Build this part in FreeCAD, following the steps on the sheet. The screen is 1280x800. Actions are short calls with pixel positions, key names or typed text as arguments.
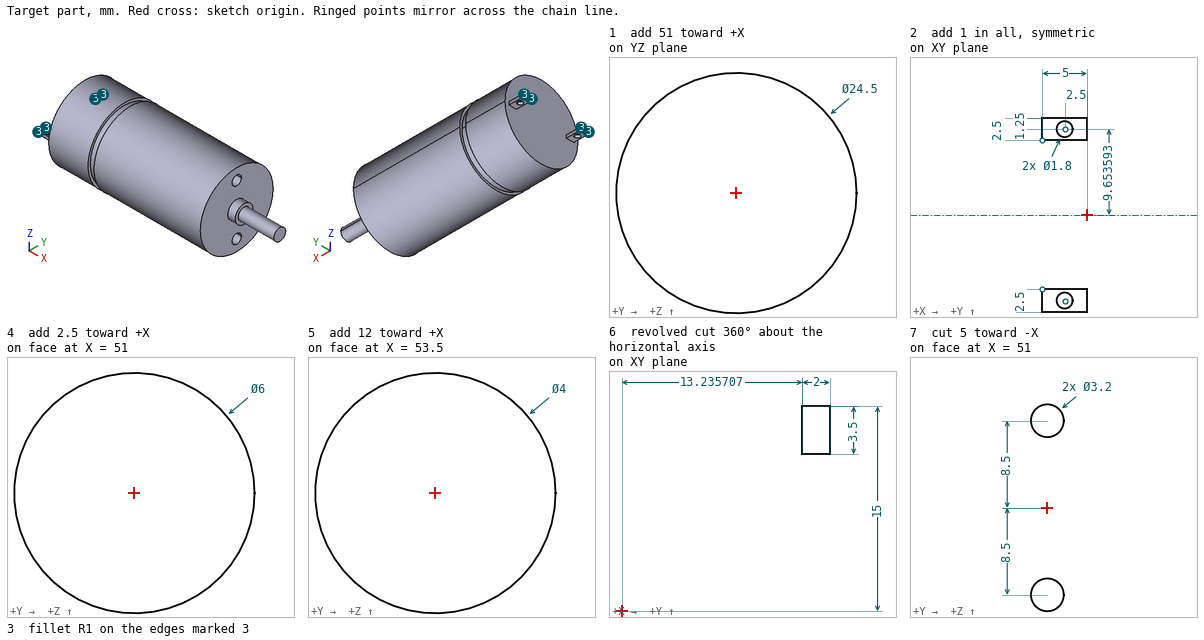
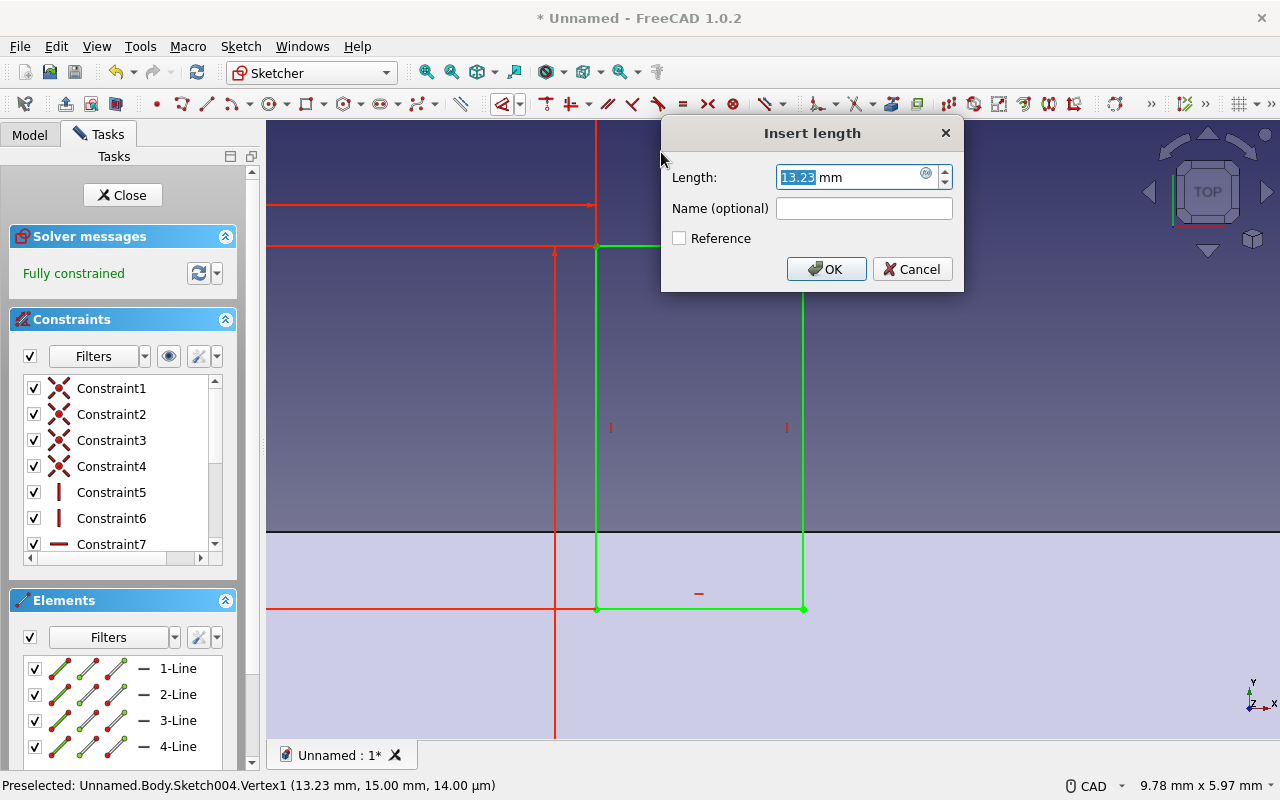
text(13.235707)
key(Return)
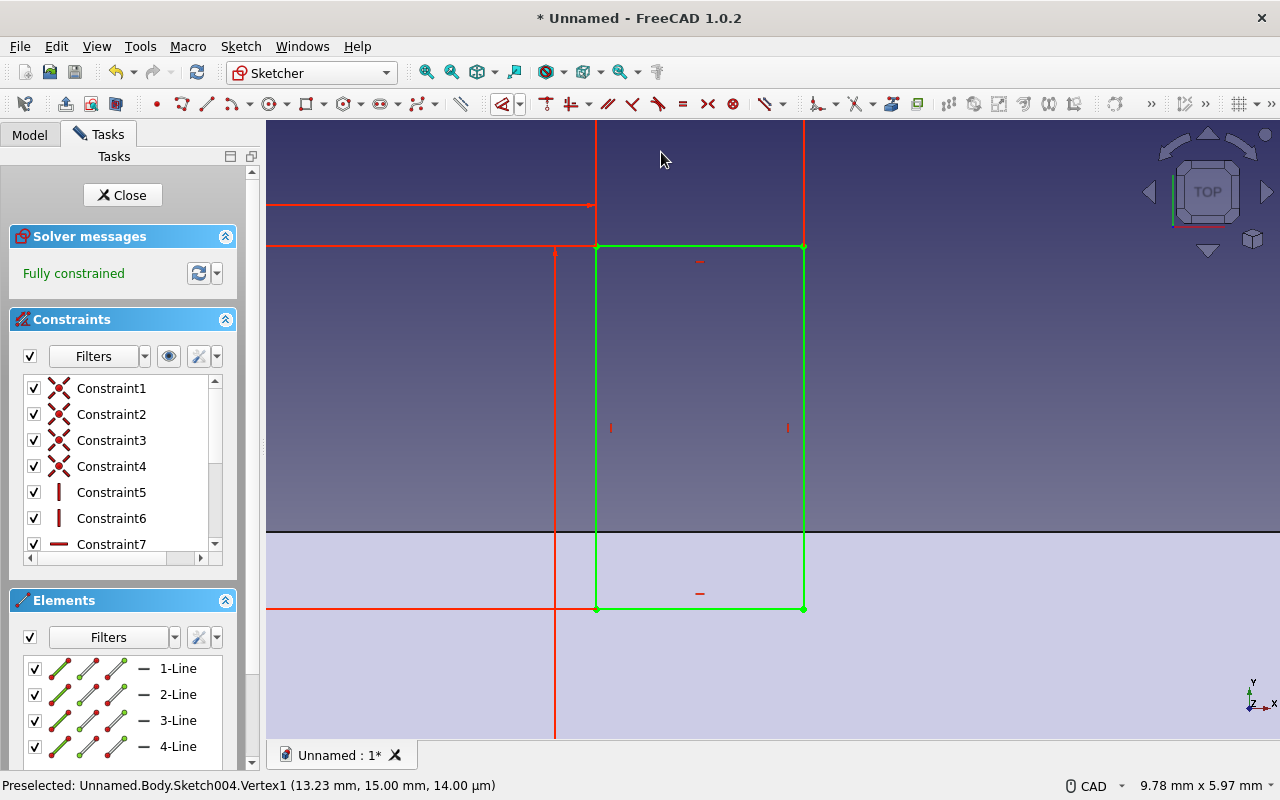
click(123, 195)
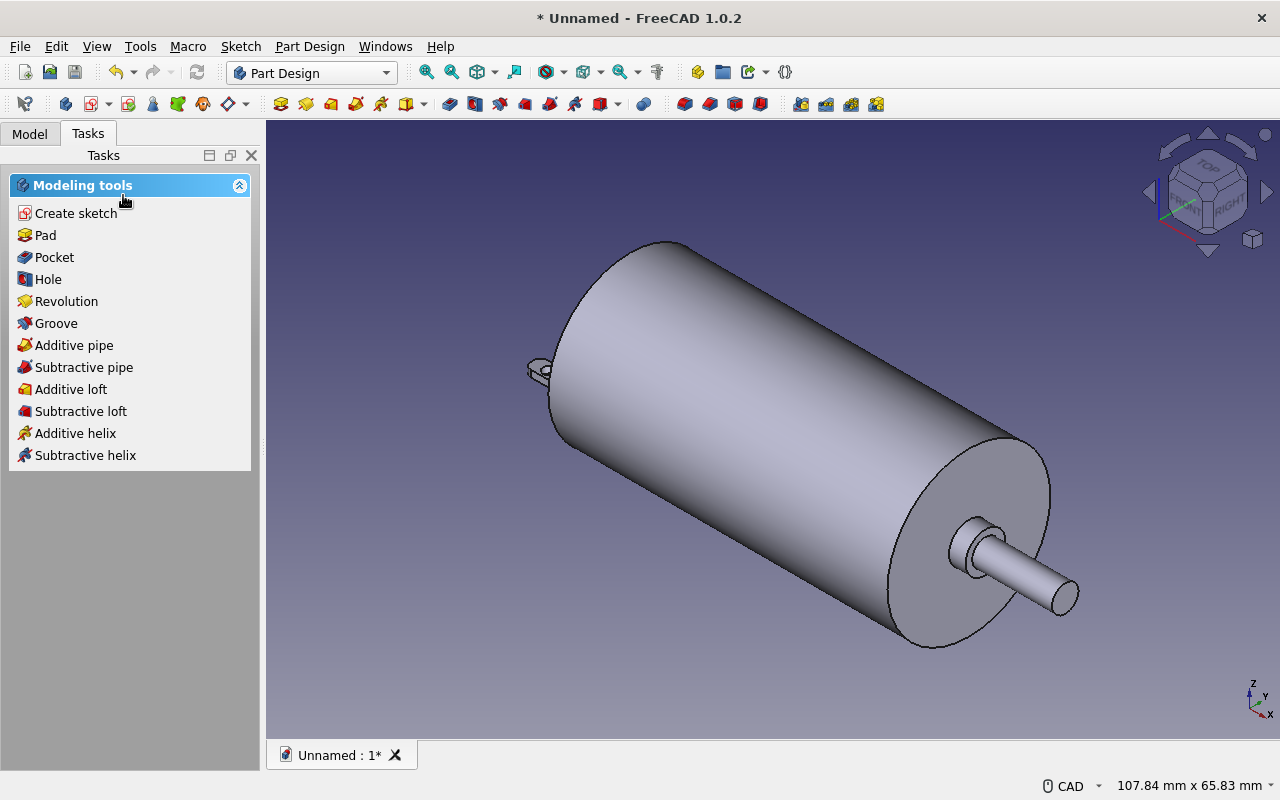
click(500, 104)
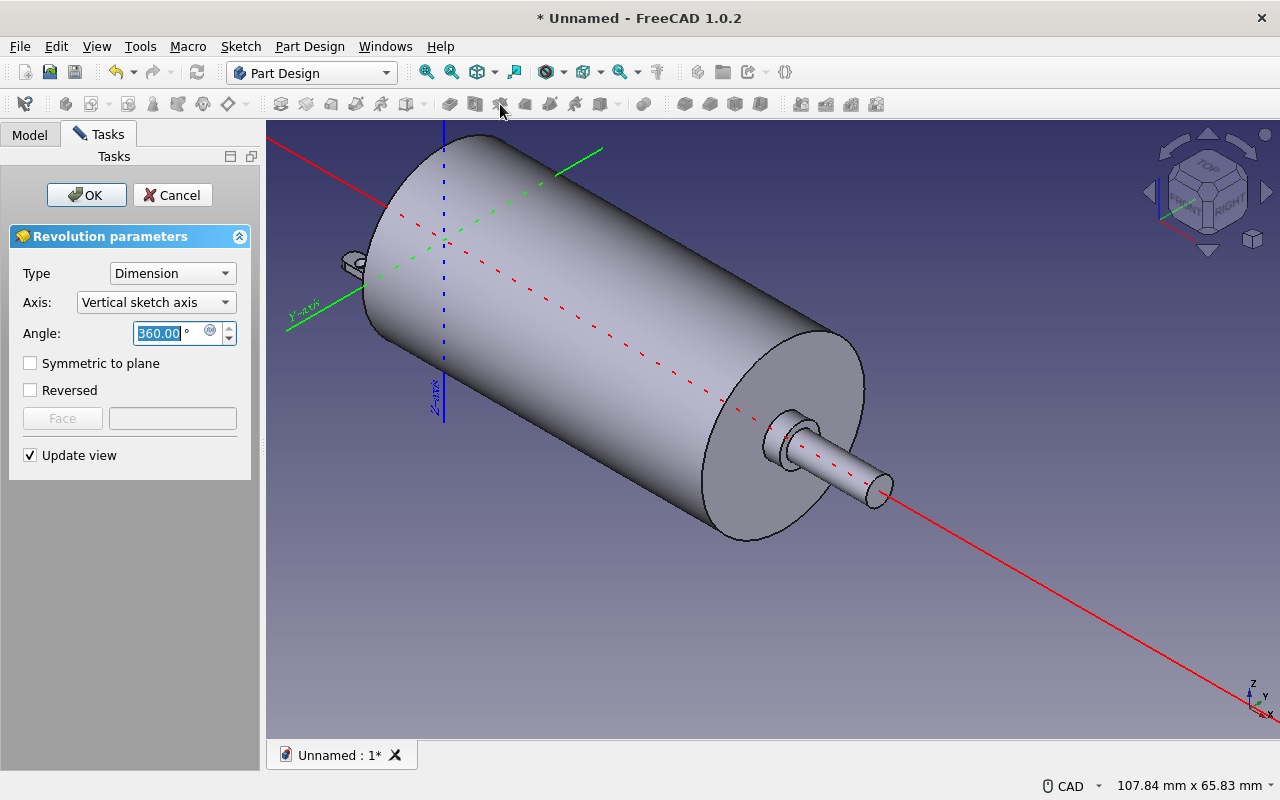
click(157, 302)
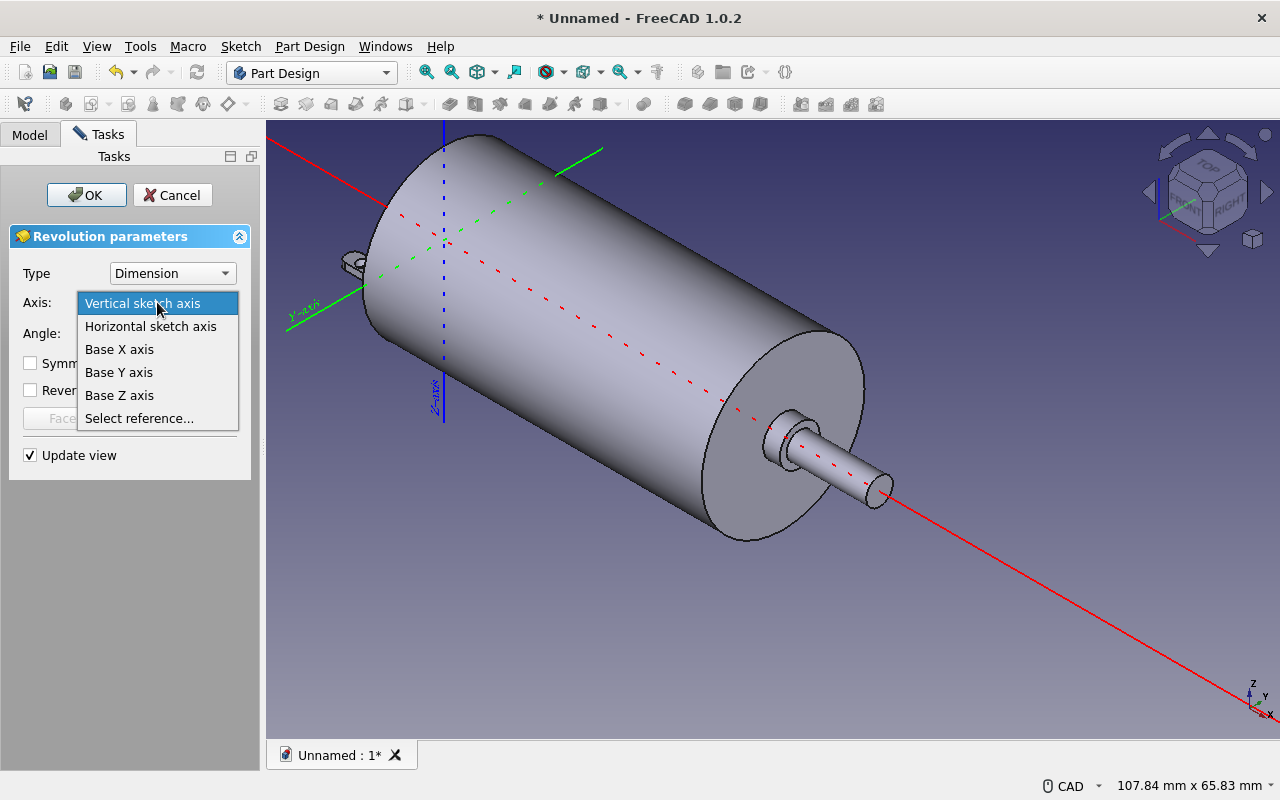
click(156, 326)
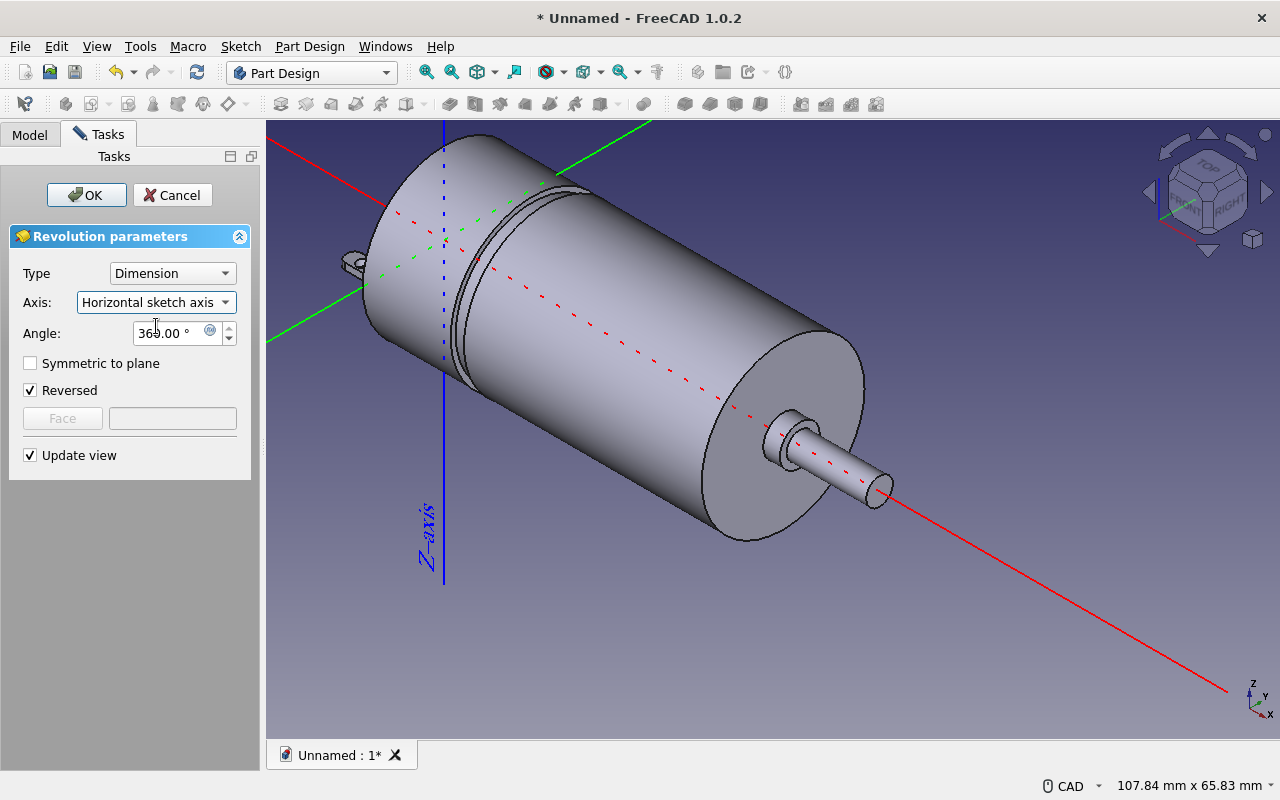
click(87, 195)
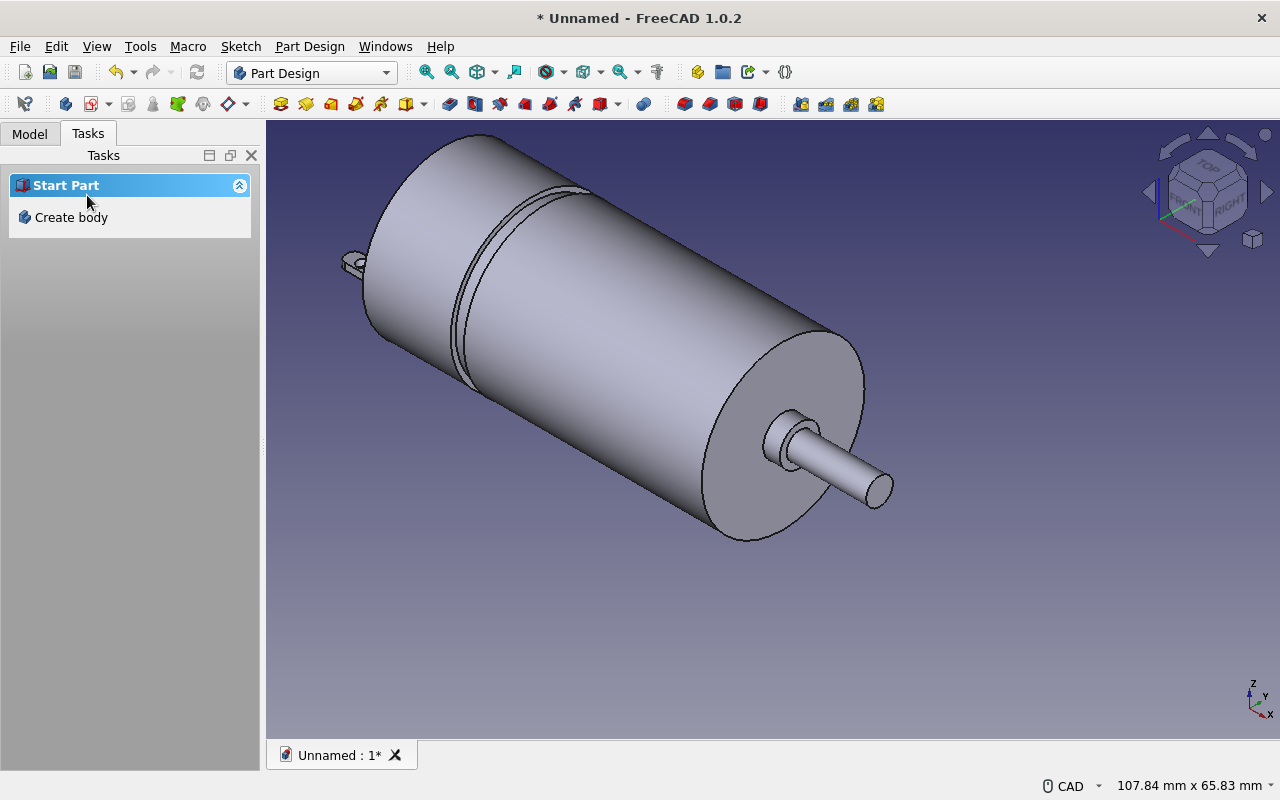
click(427, 72)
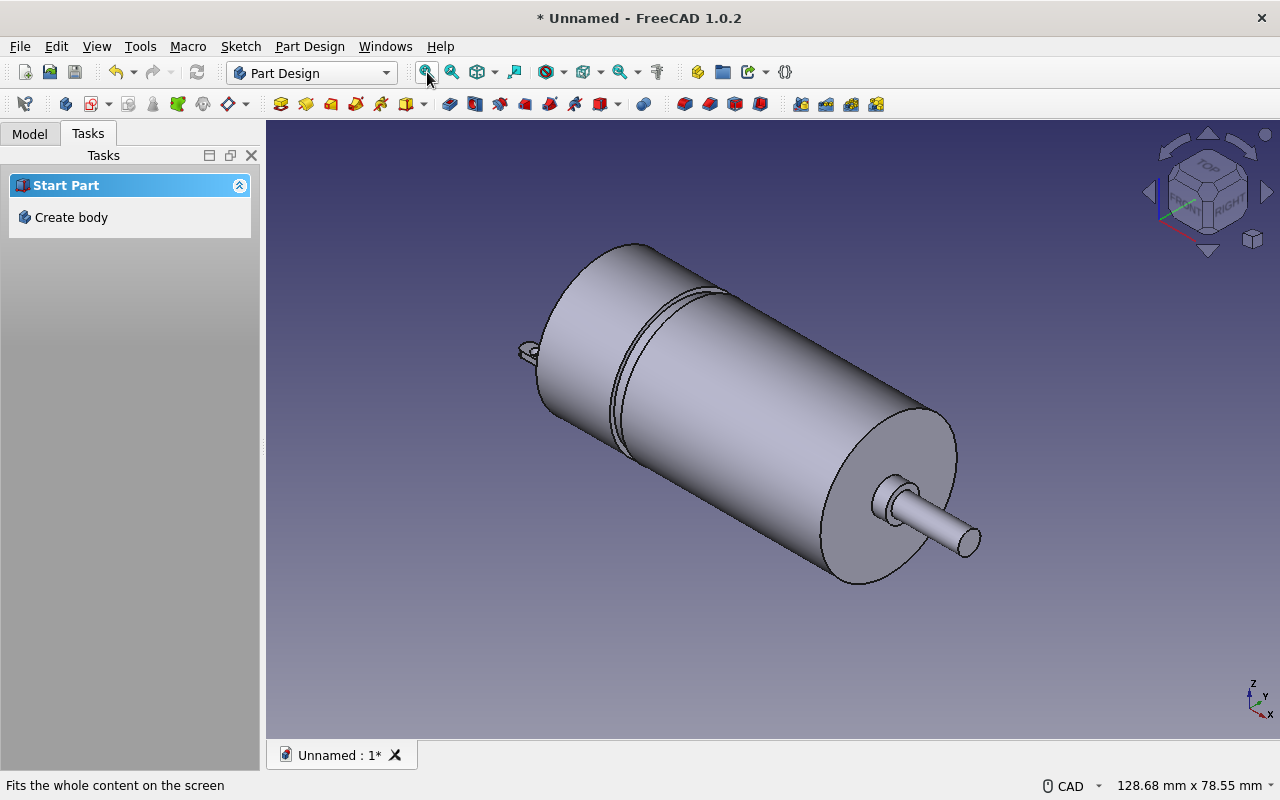
click(869, 461)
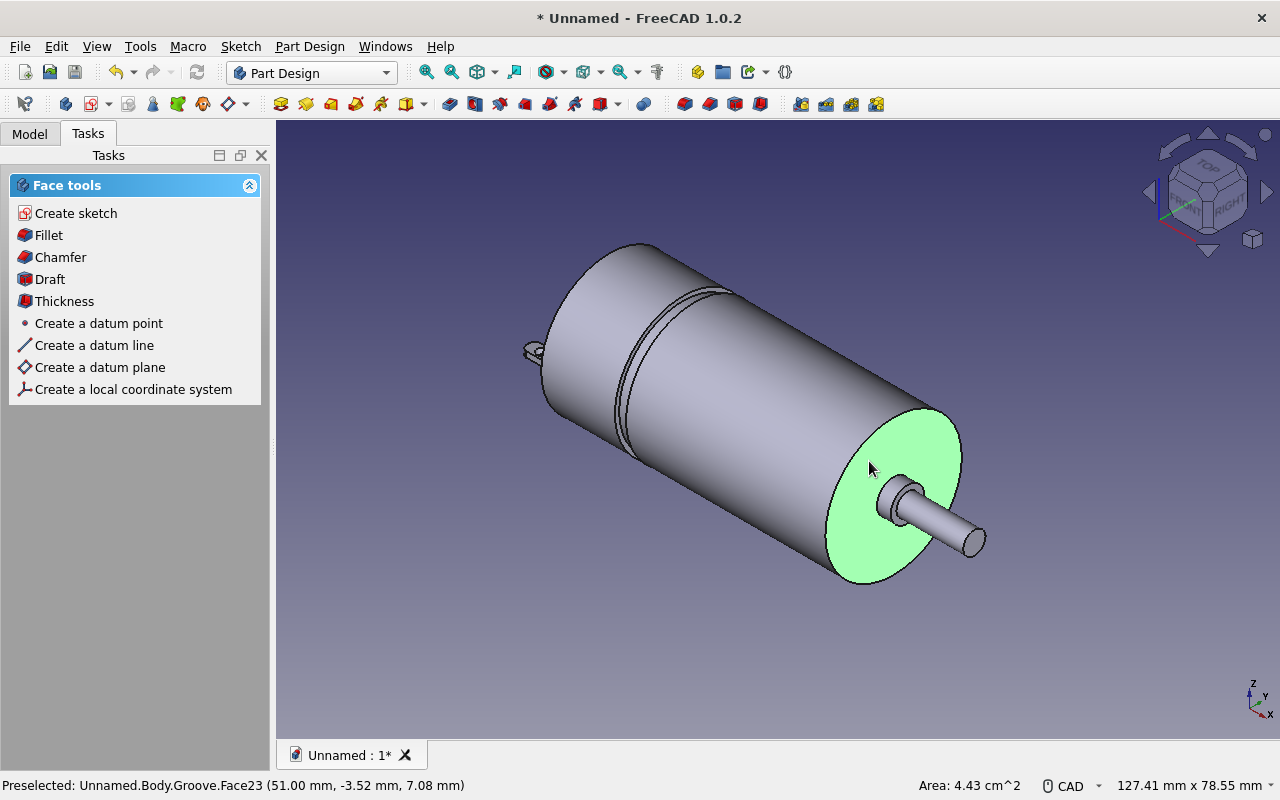
click(90, 104)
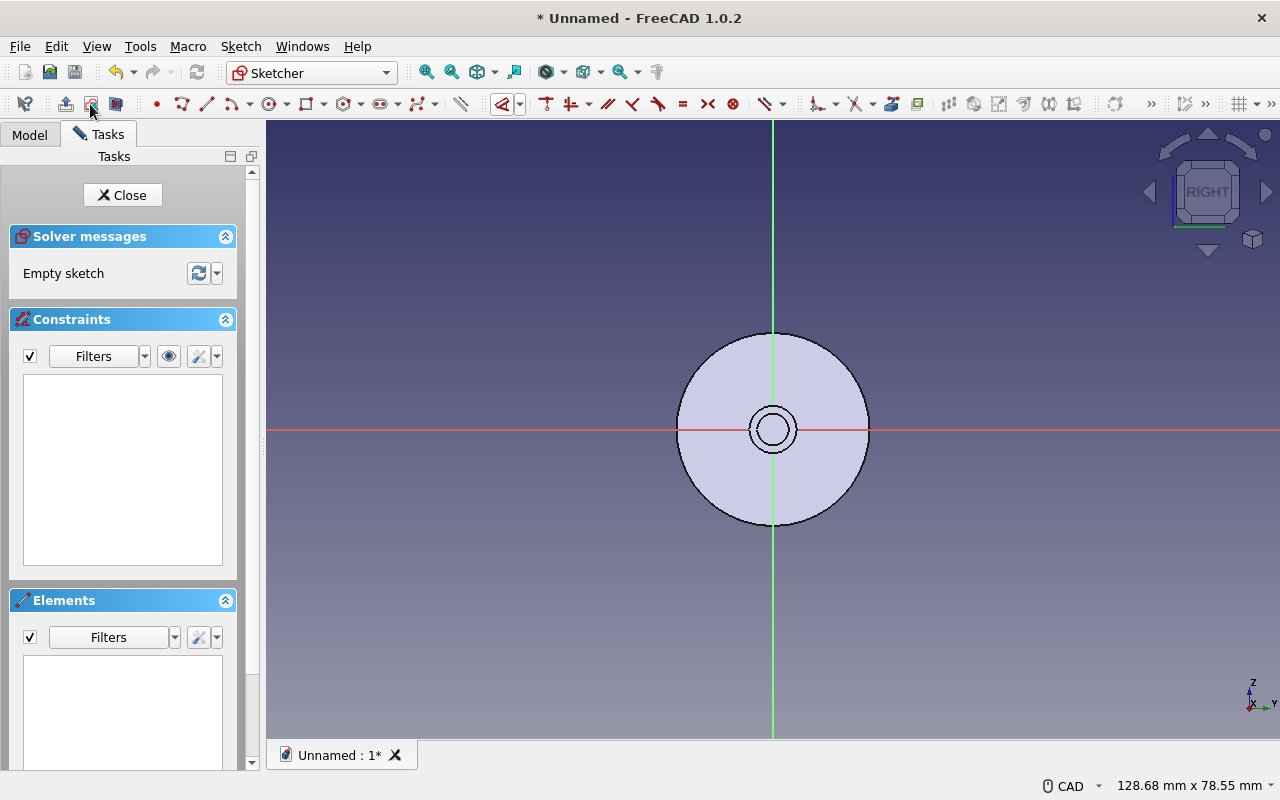
click(116, 104)